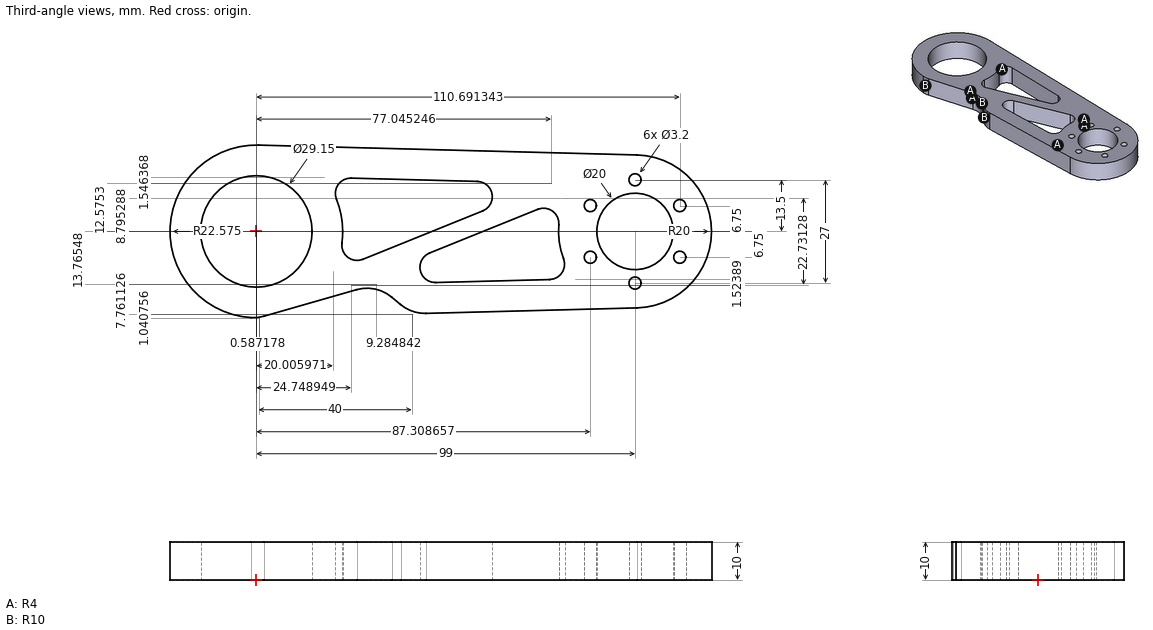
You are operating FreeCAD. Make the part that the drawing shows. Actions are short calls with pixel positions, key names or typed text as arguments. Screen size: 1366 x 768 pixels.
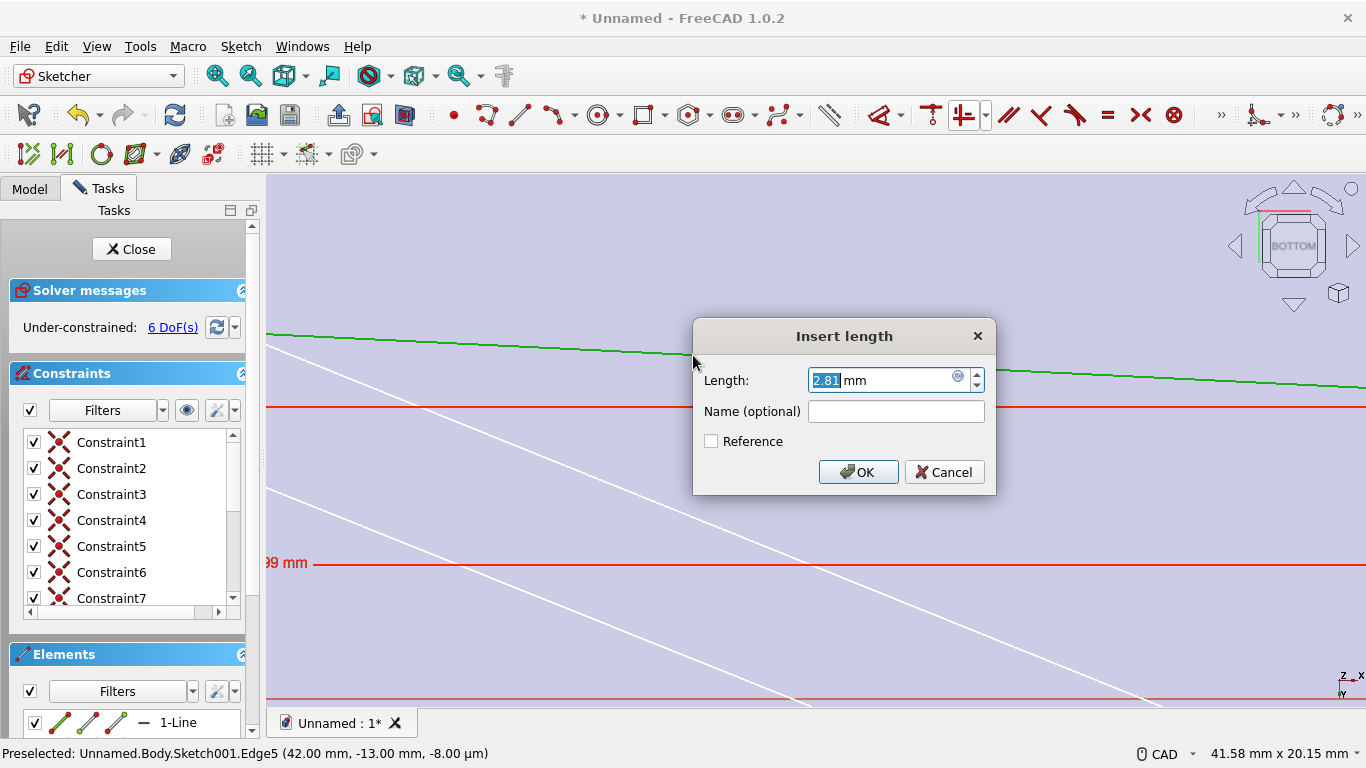
text(1.52389)
key(Return)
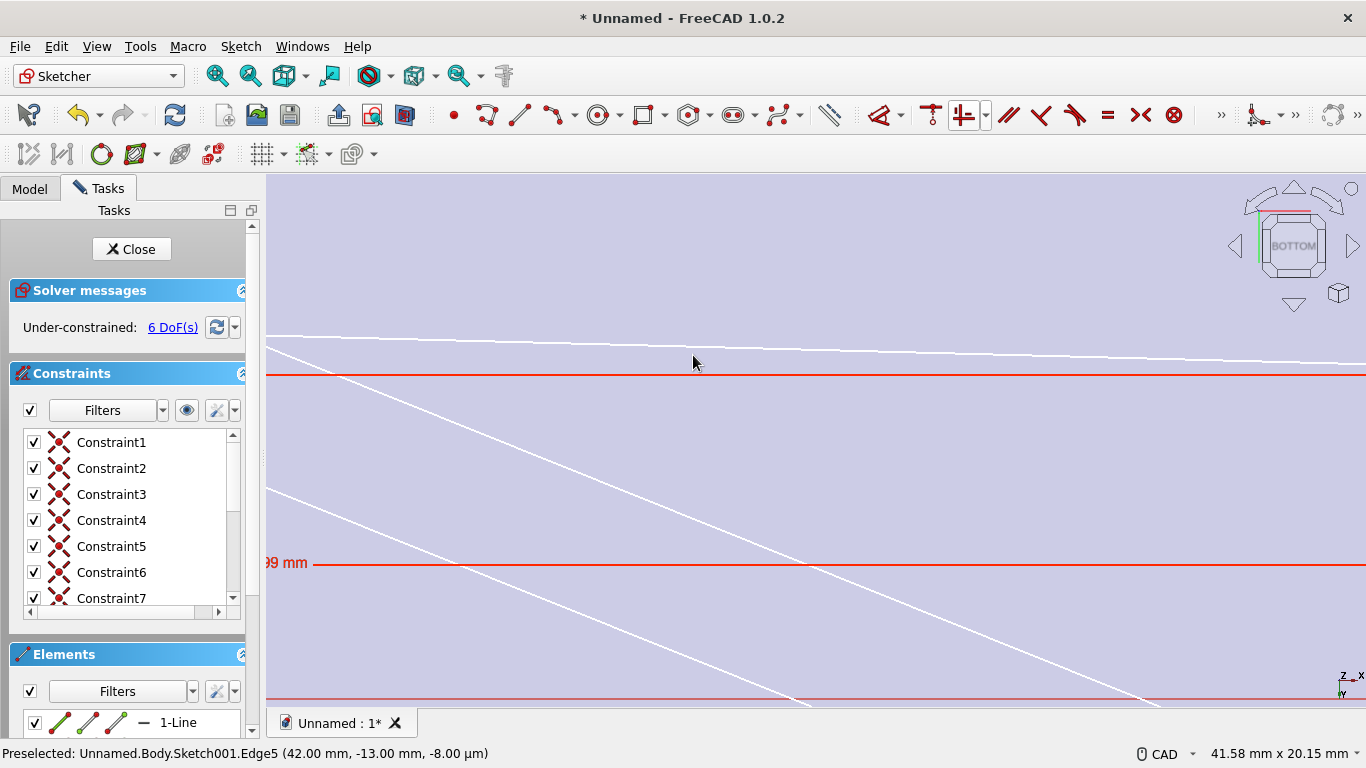
scroll(775, 328, down, 6)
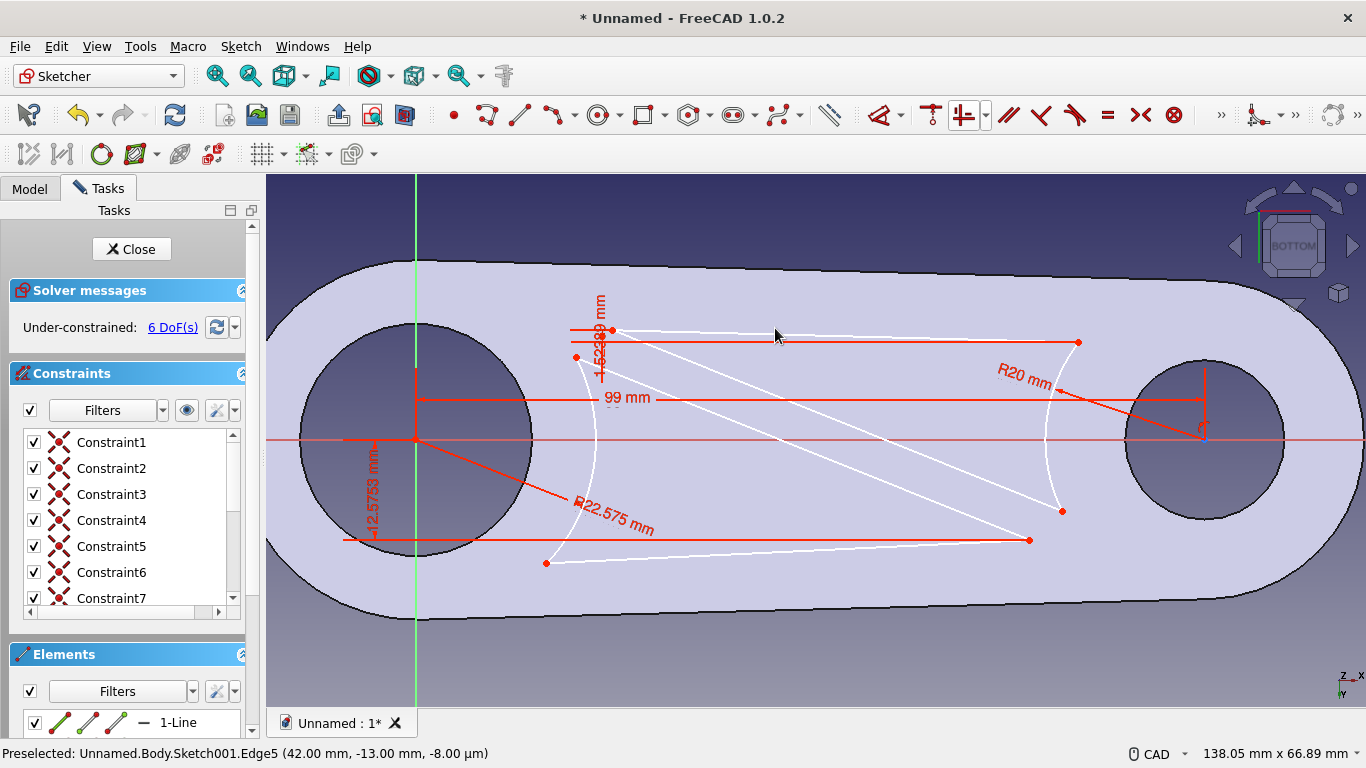
click(1062, 511)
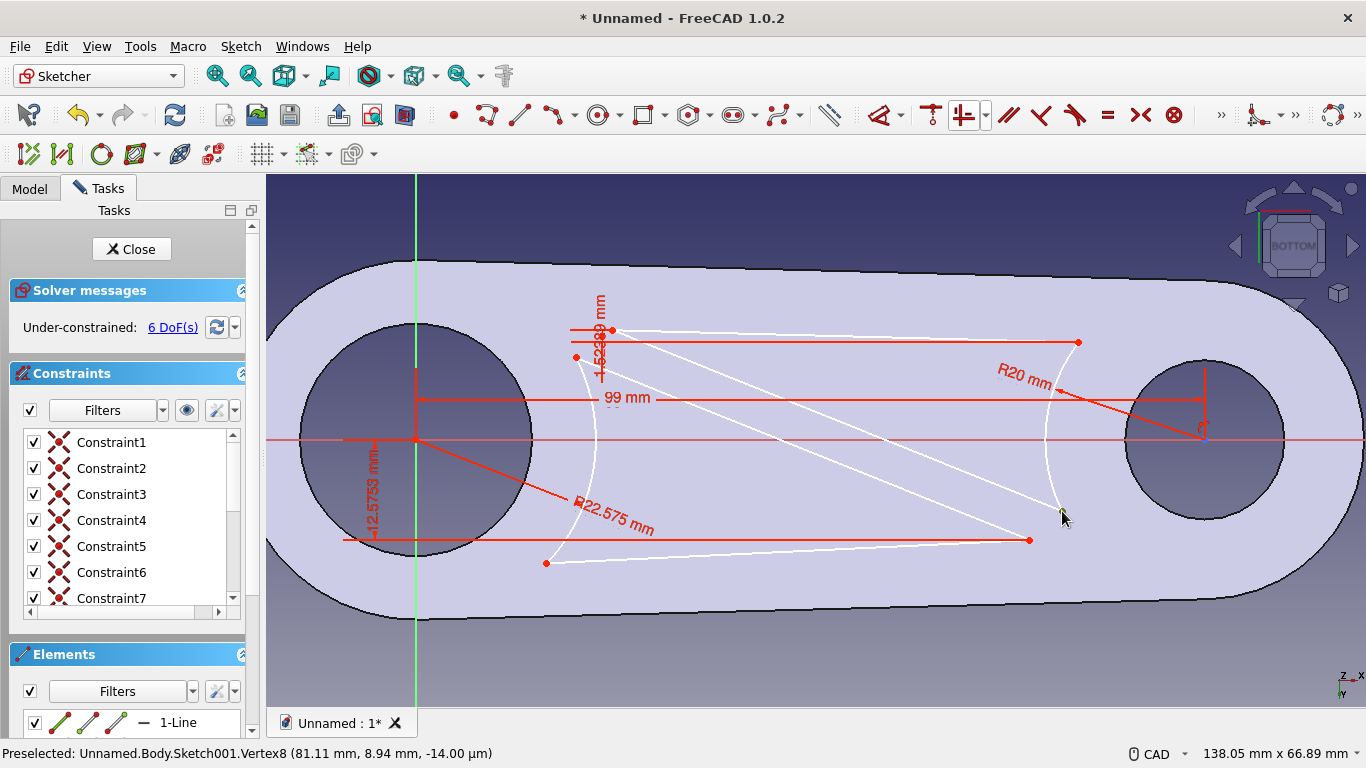
click(900, 116)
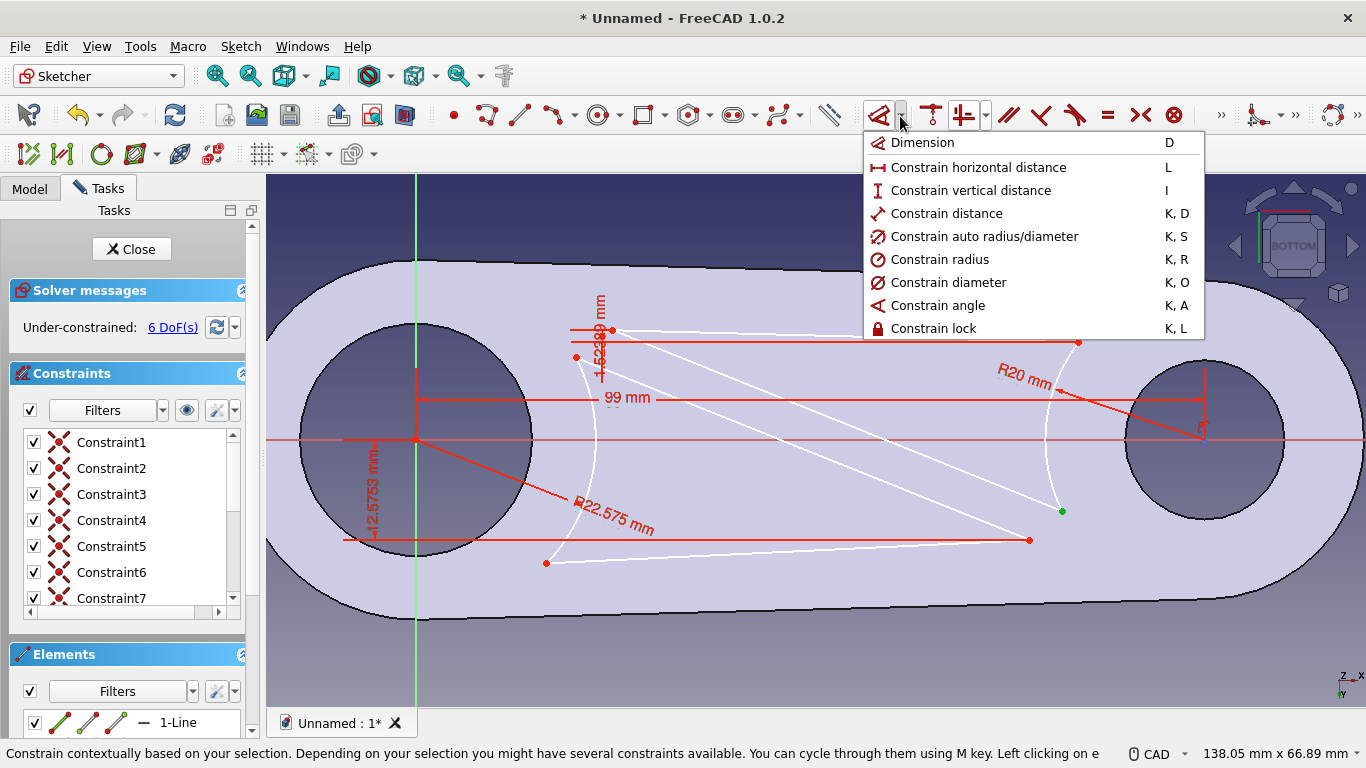
click(1034, 190)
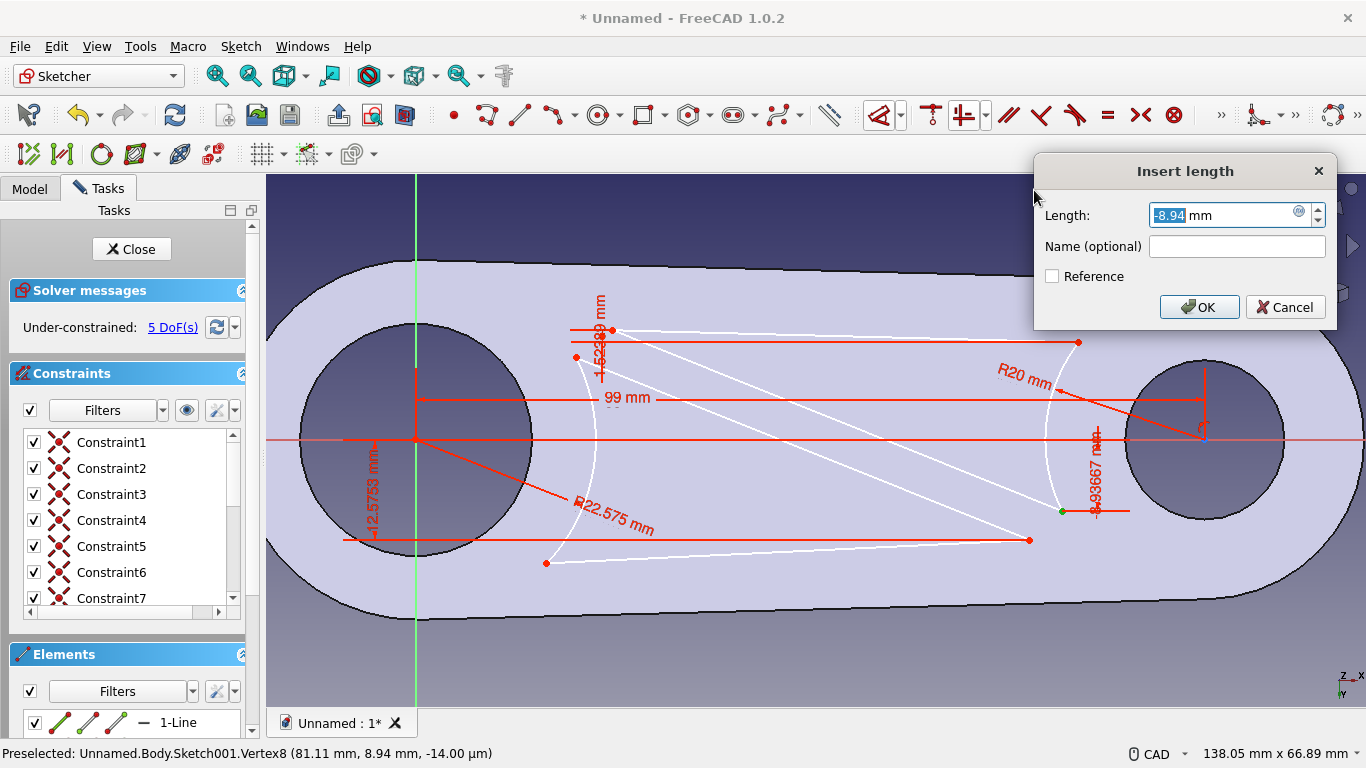
text(-8.795288)
key(Return)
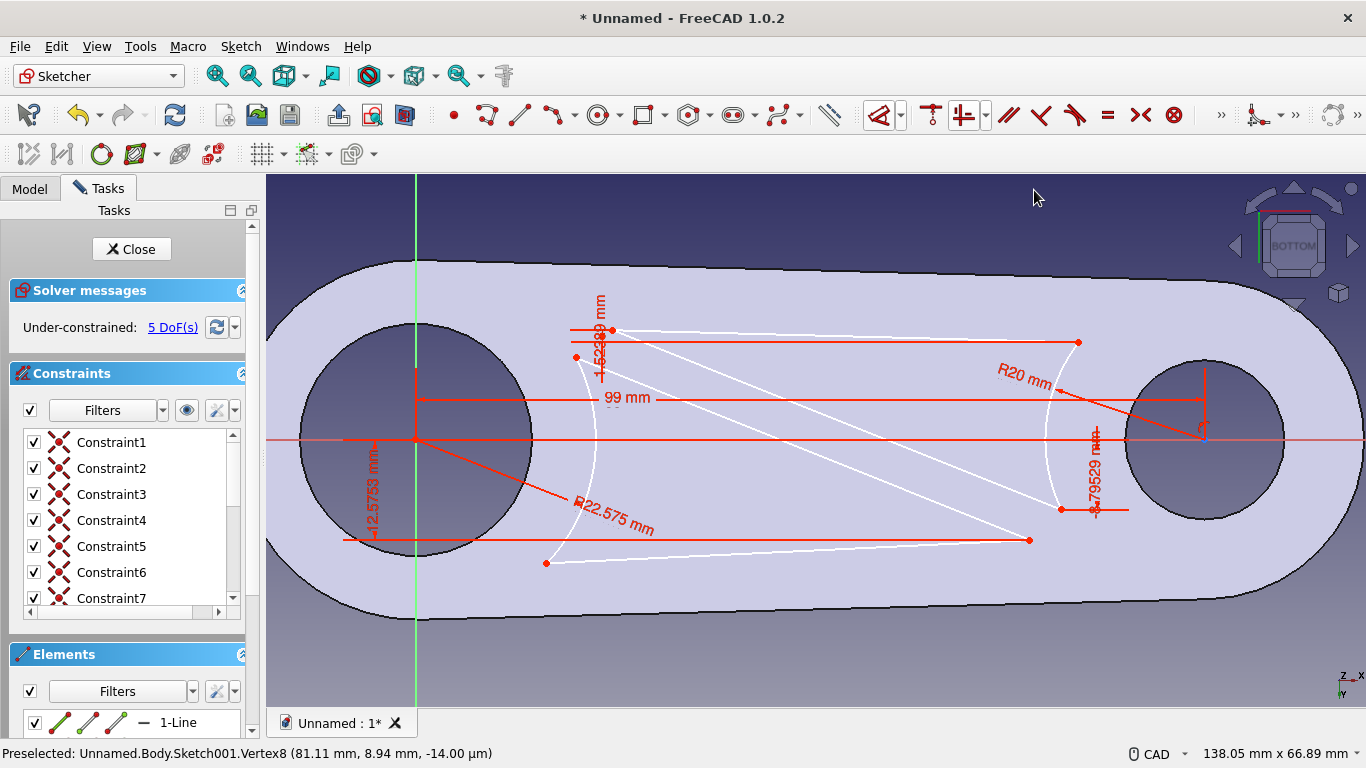
scroll(885, 547, up, 6)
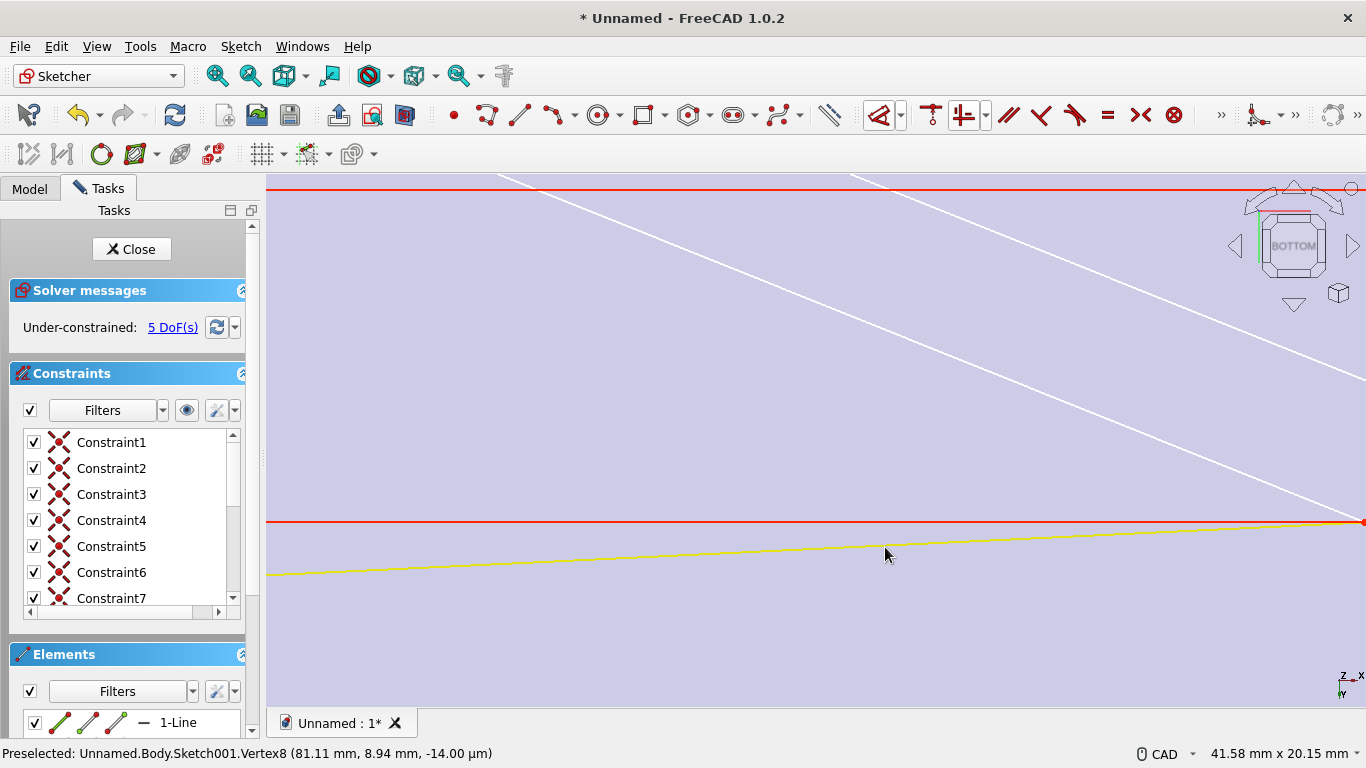
click(884, 546)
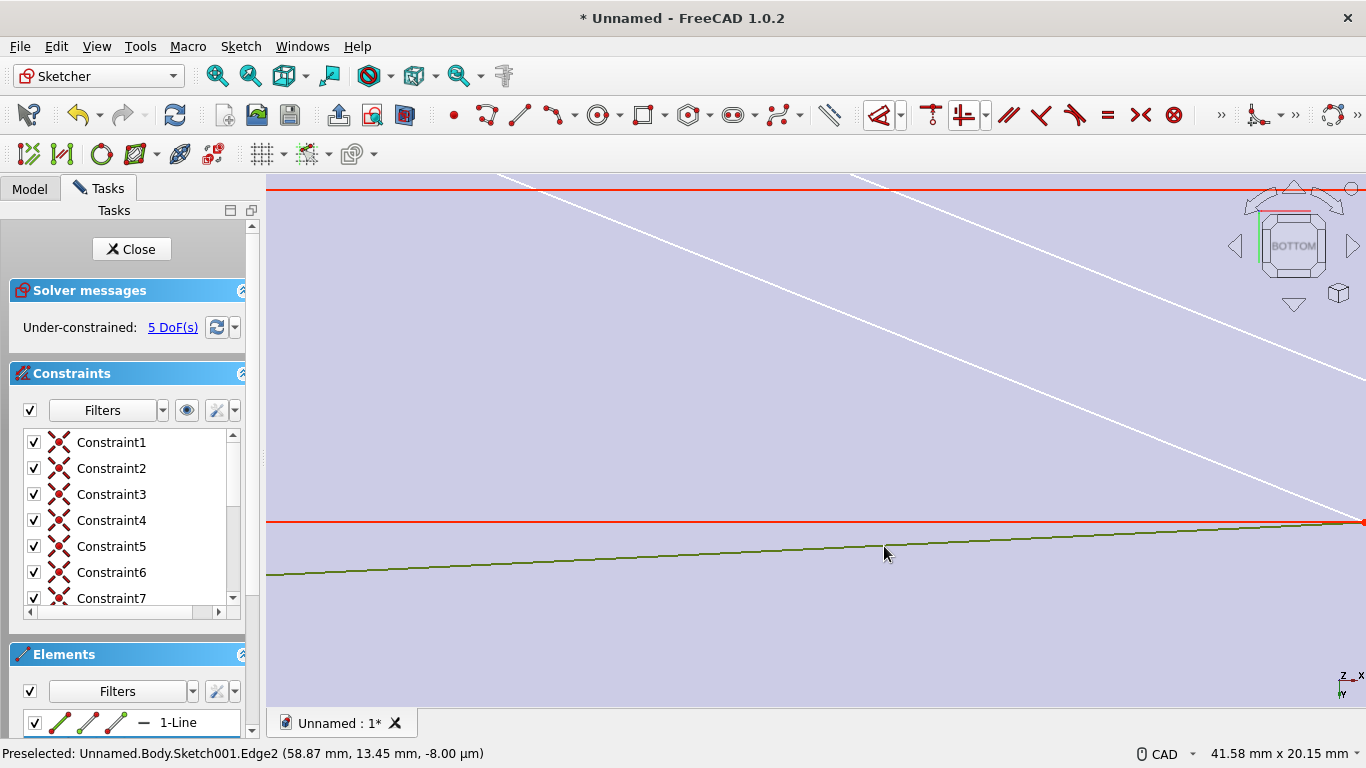
key(i)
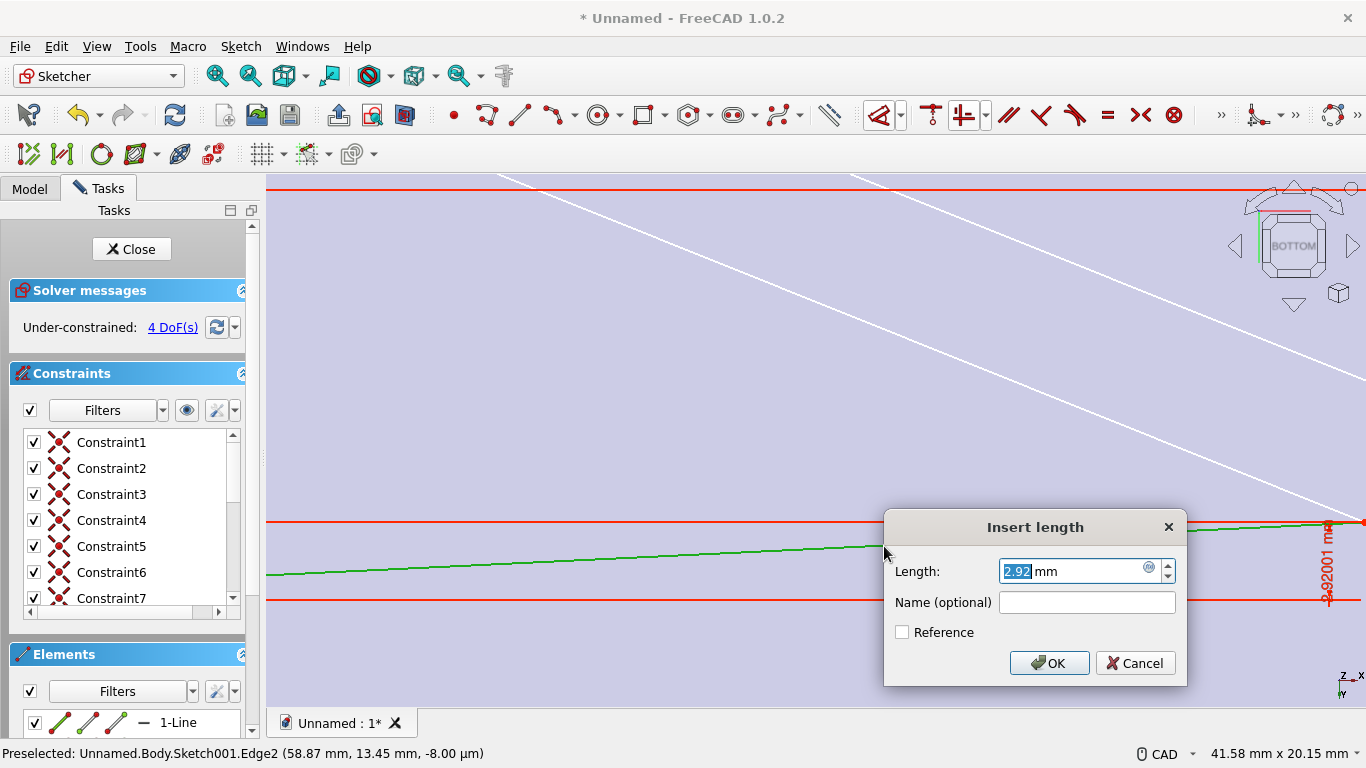
text(1.546368)
key(Return)